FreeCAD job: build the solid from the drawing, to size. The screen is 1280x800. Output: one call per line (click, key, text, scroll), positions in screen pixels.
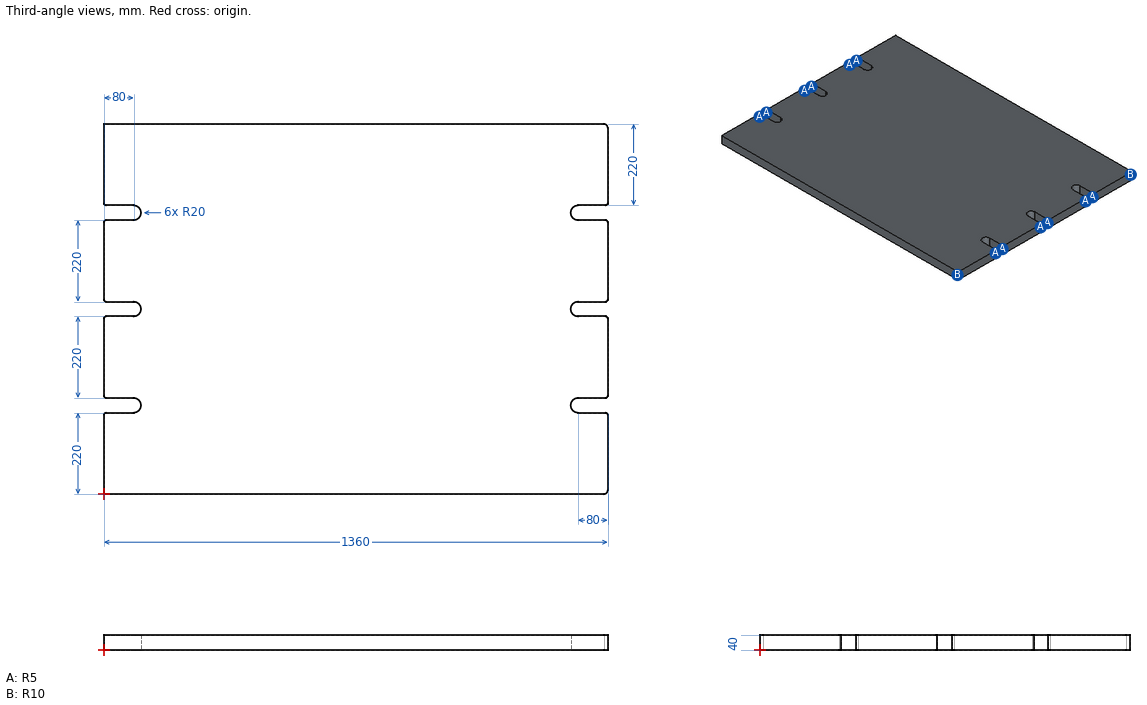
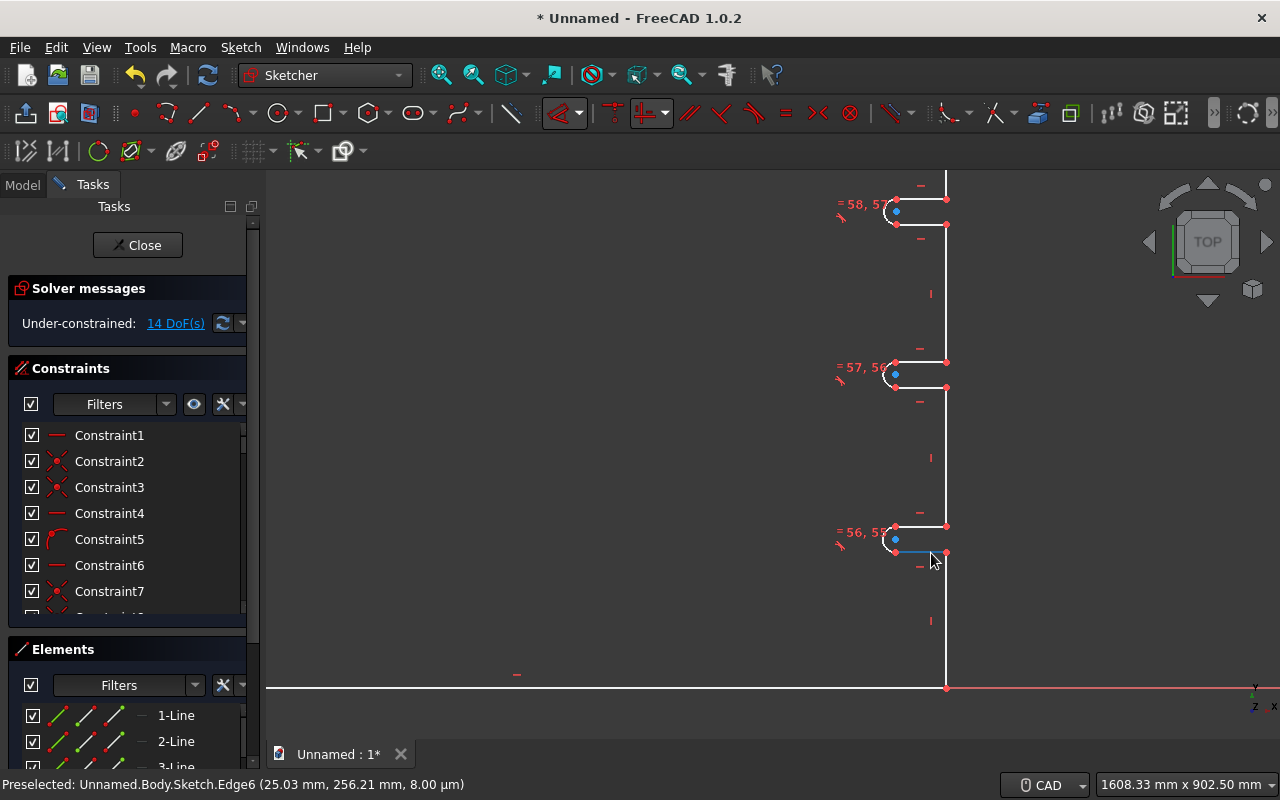
click(931, 552)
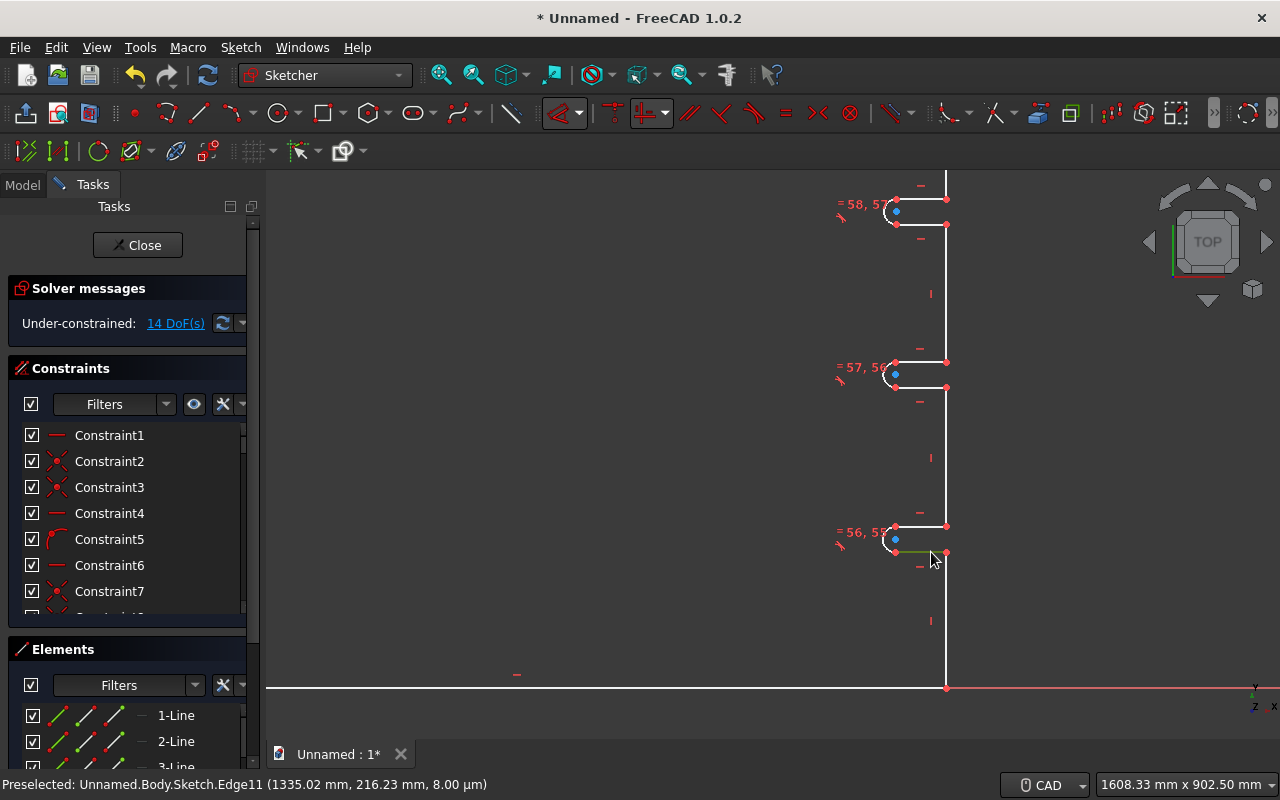
click(582, 114)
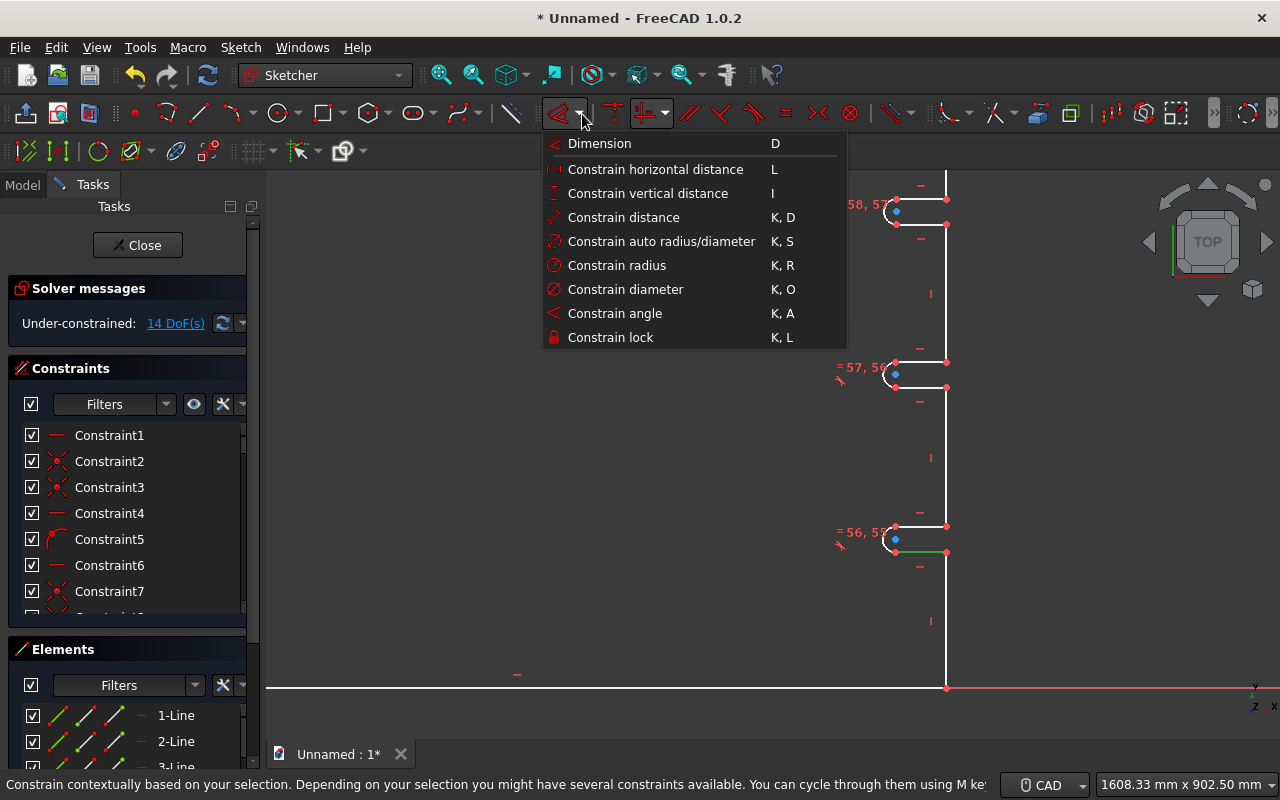
click(695, 169)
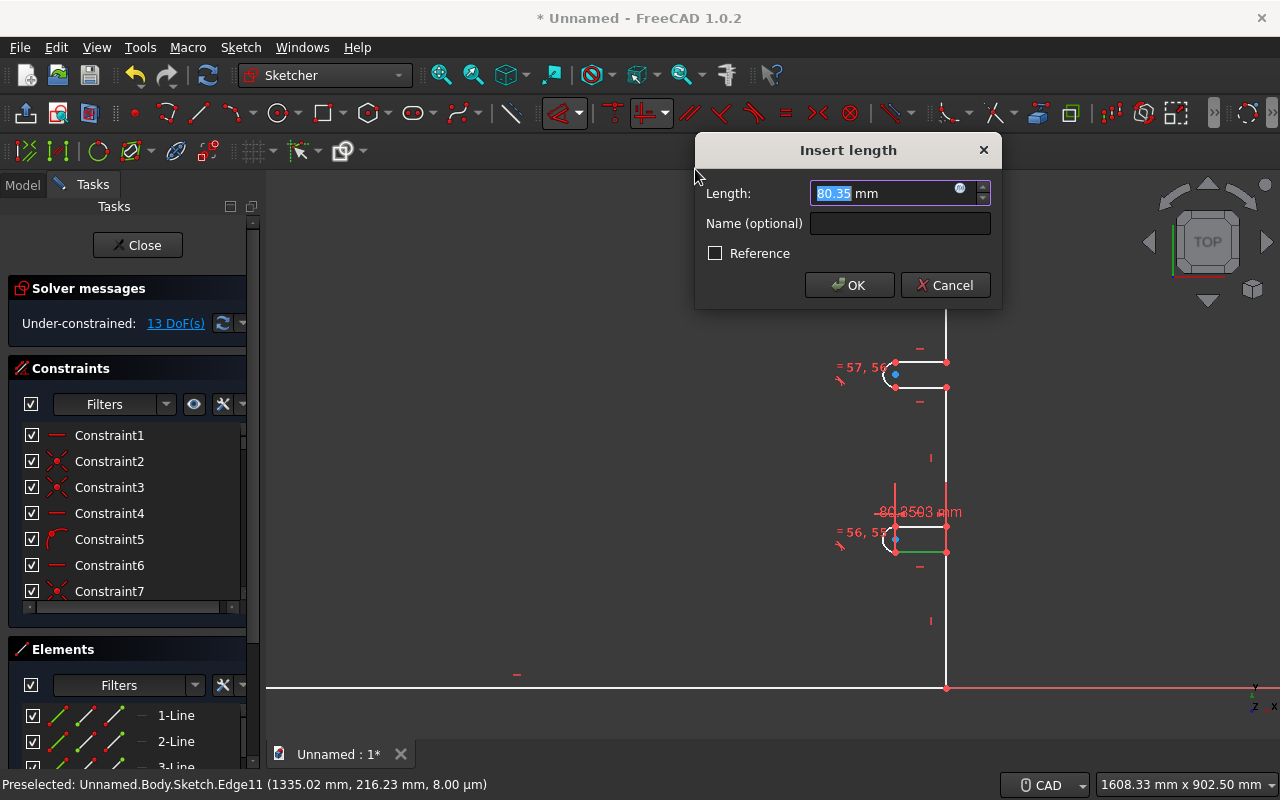
text(80)
key(Return)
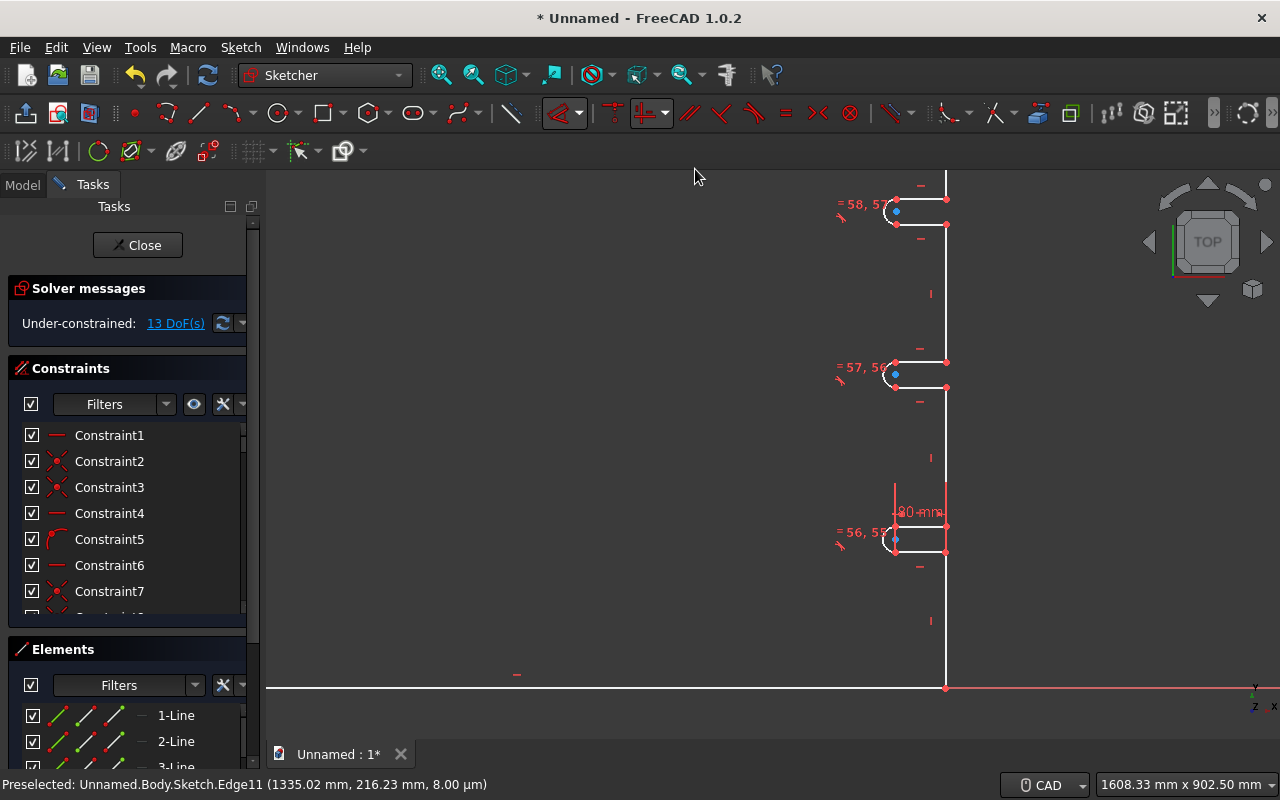
click(911, 527)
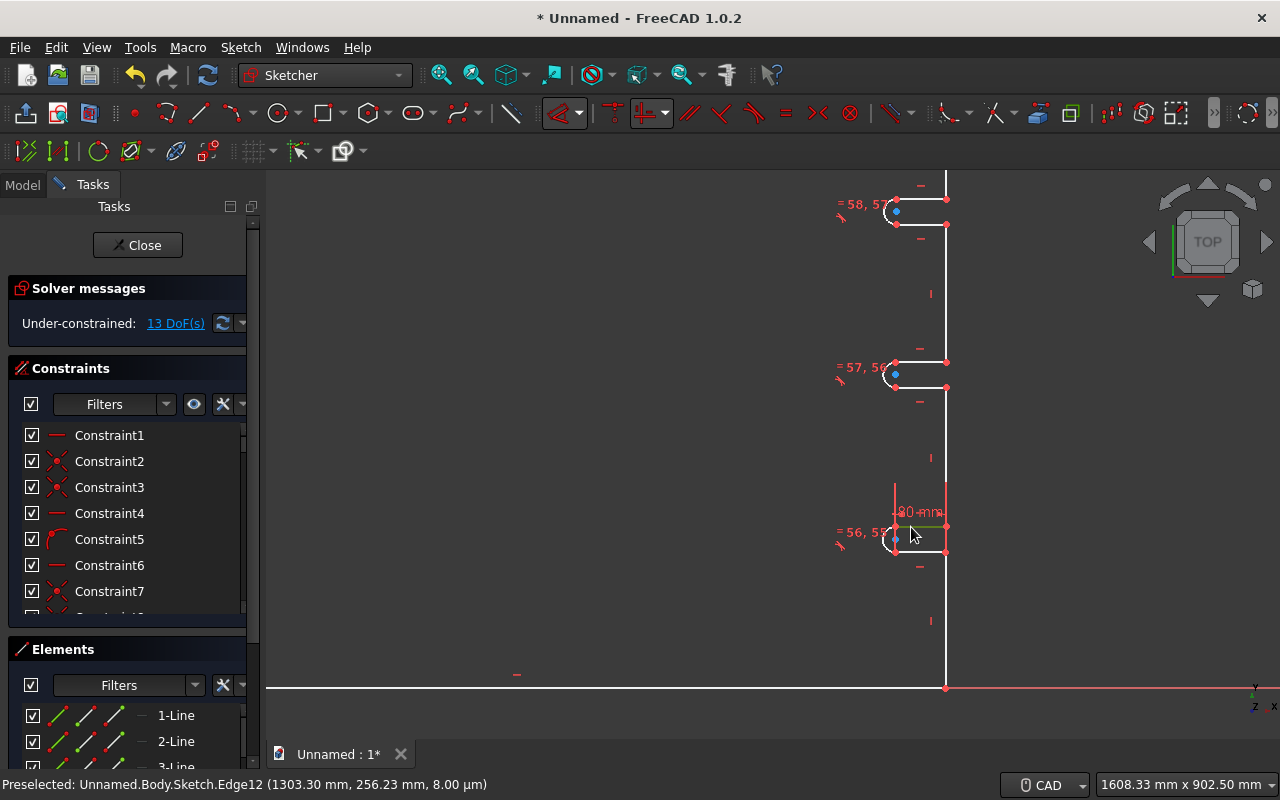
key(l)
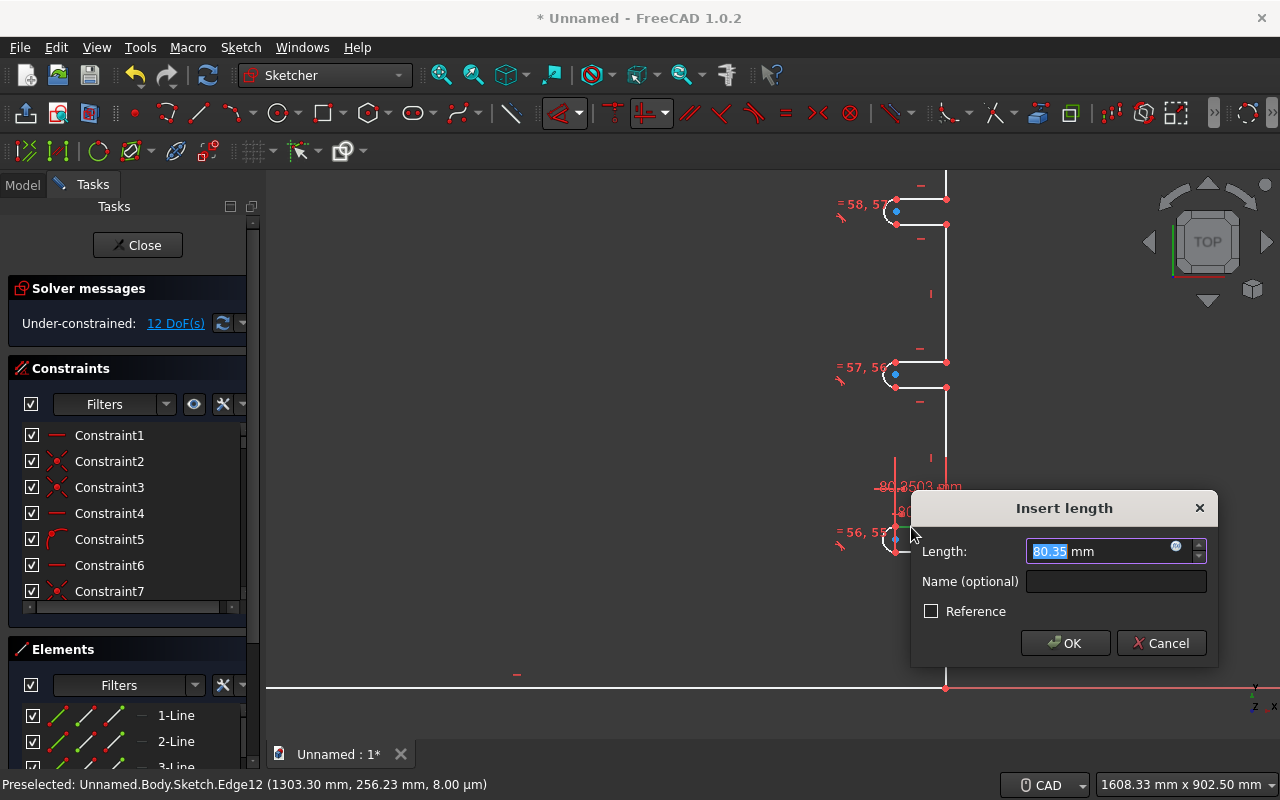
text(80)
key(Return)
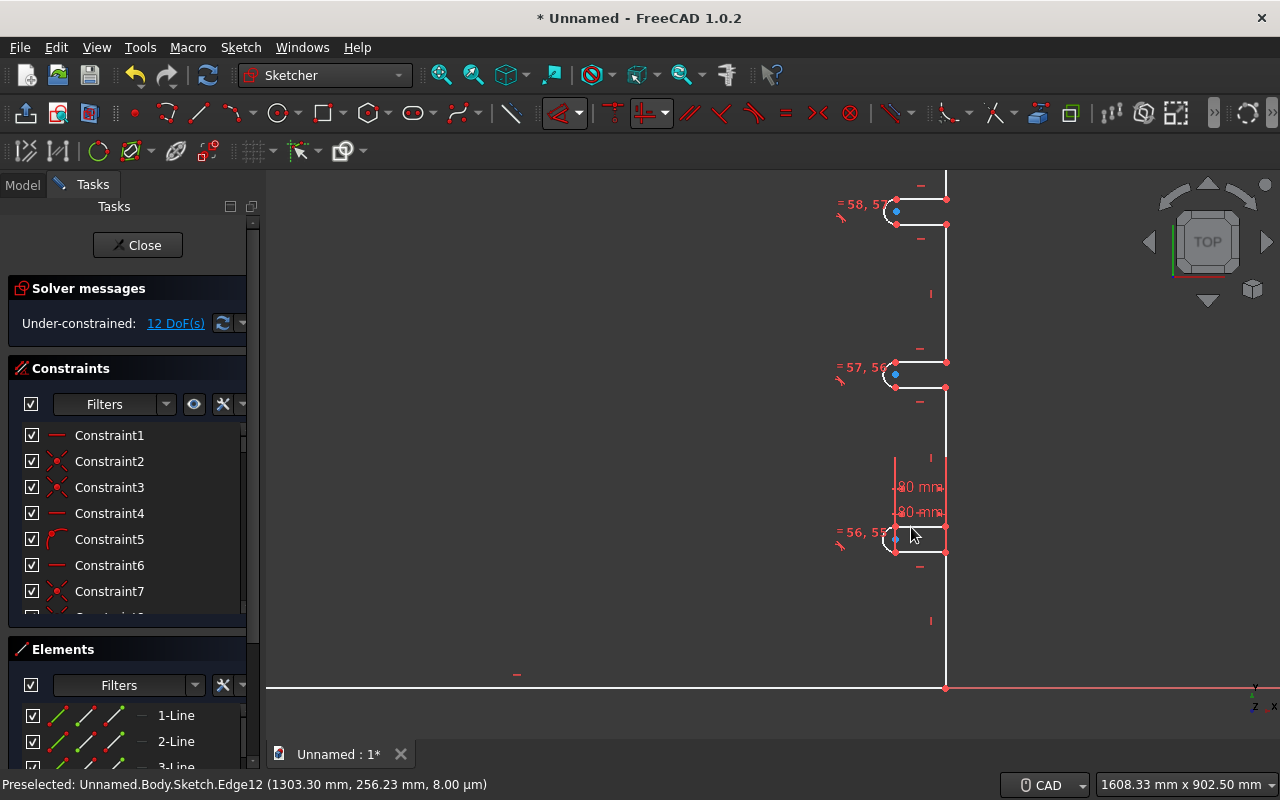
click(931, 388)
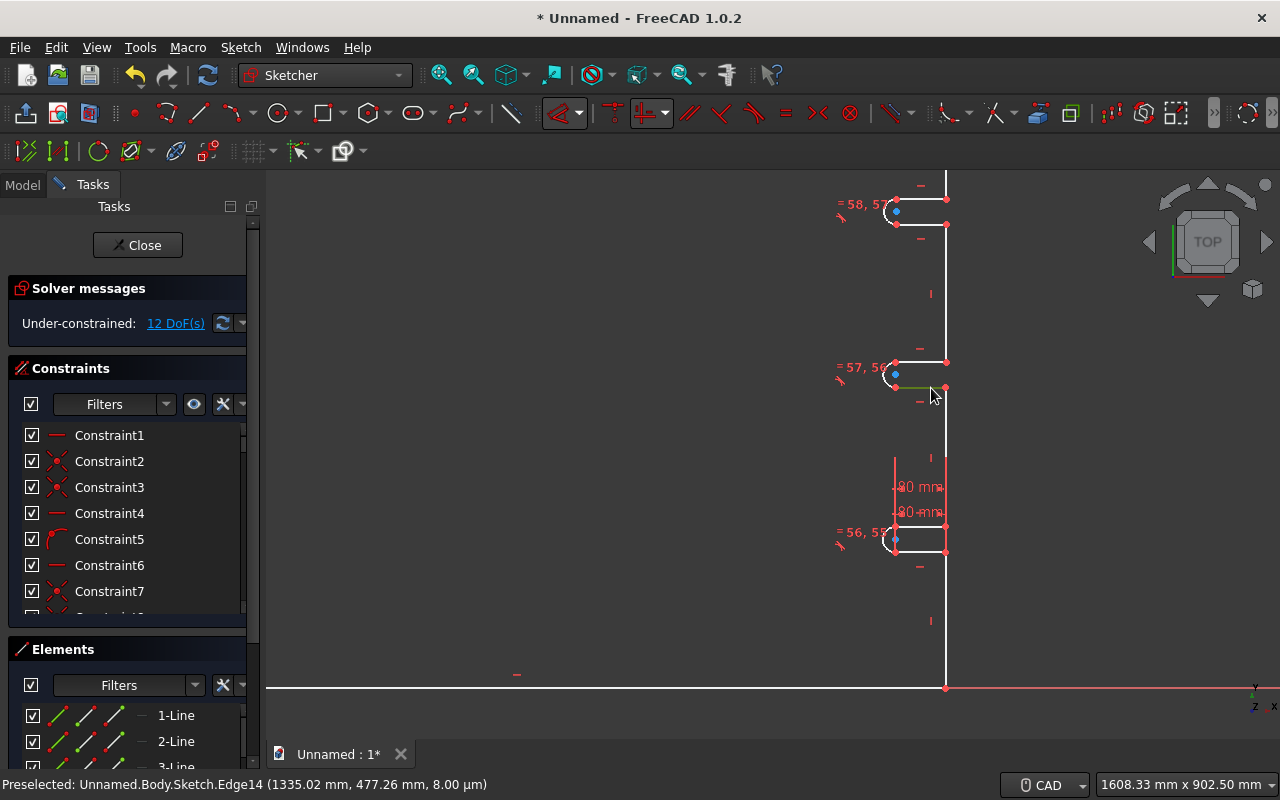
click(582, 114)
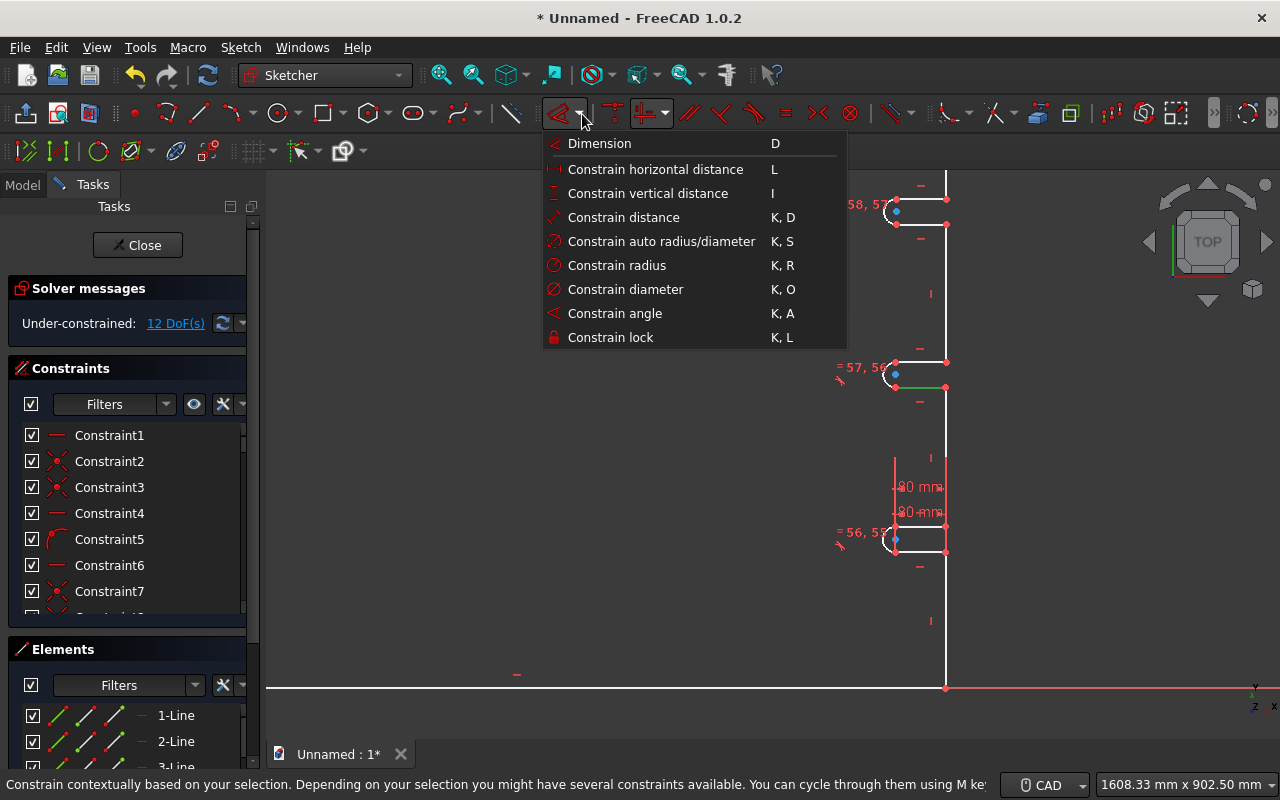
click(695, 169)